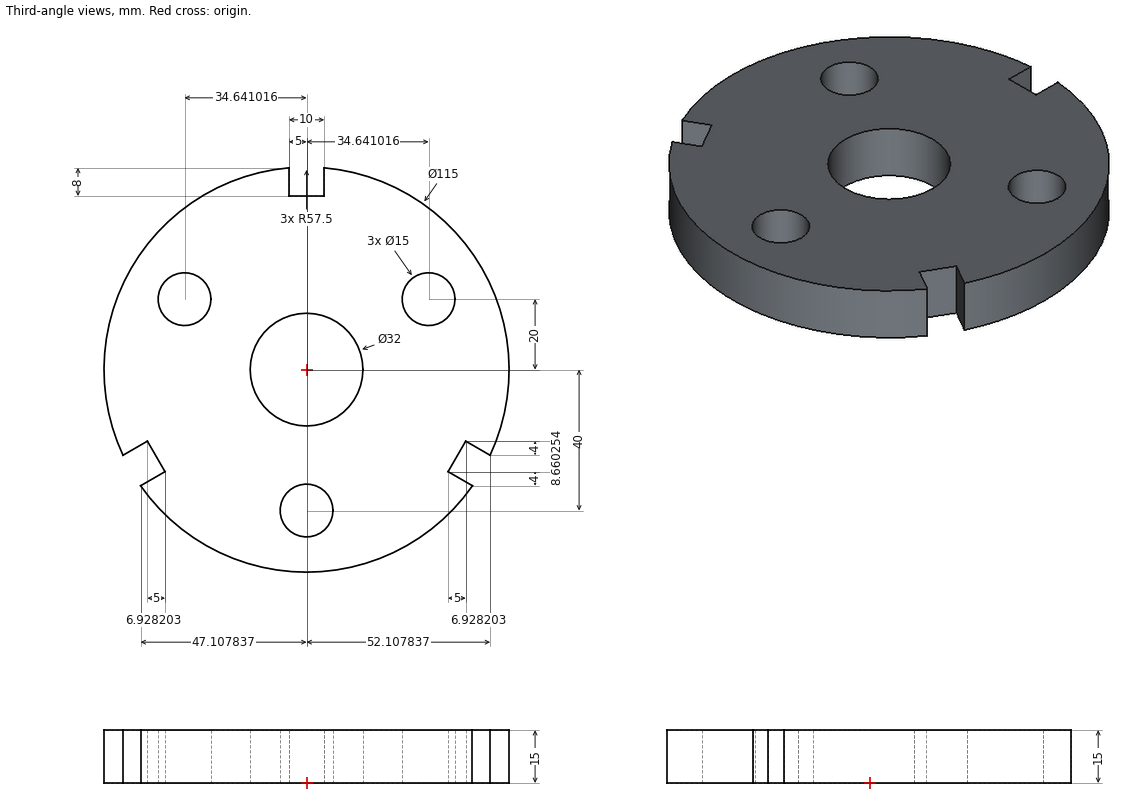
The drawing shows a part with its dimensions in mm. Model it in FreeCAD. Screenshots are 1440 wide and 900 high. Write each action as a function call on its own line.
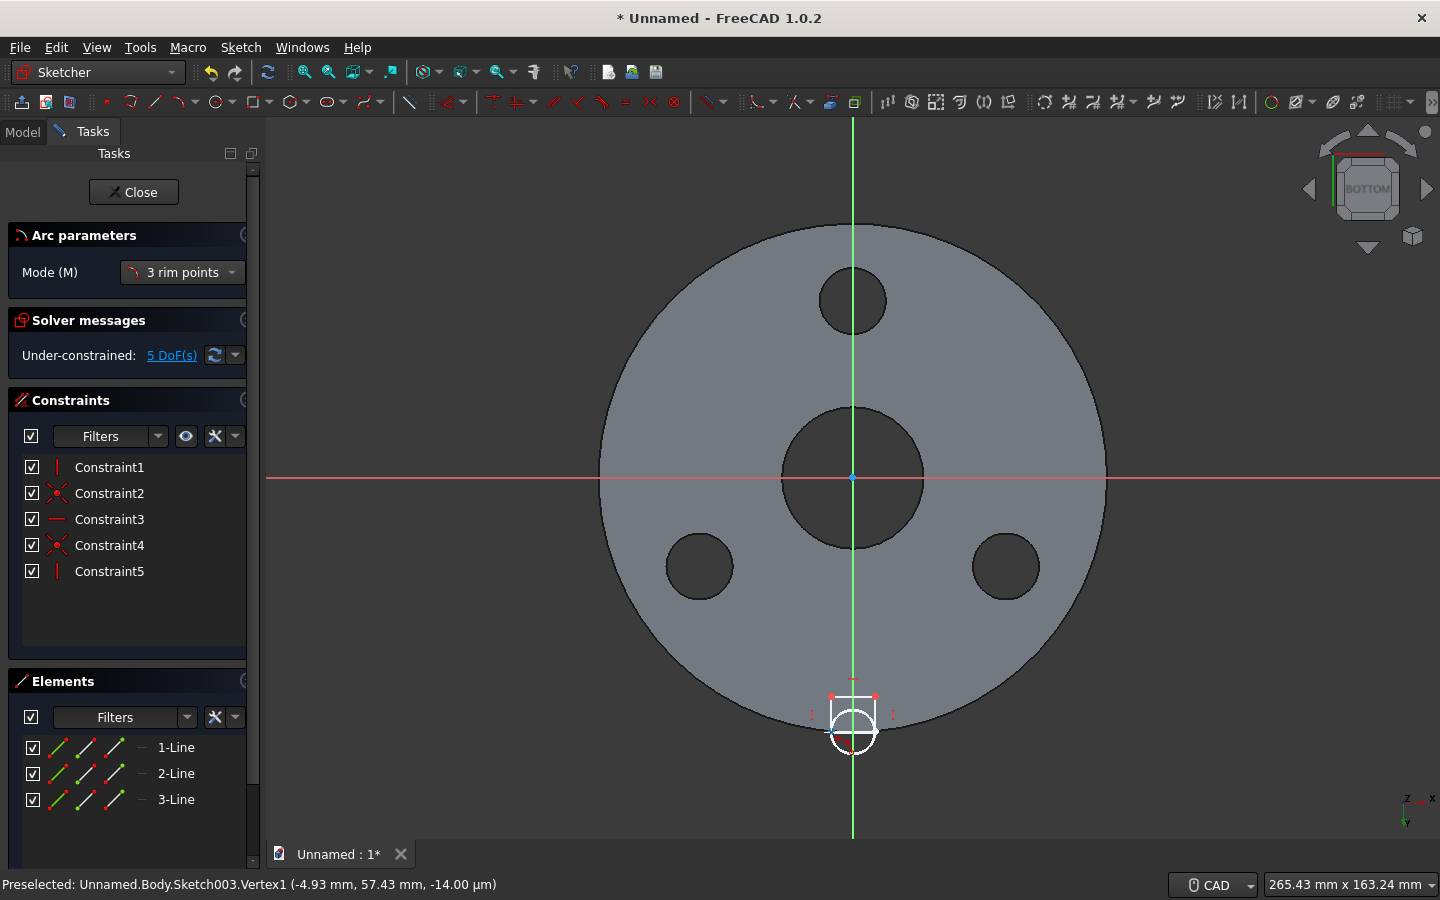
scroll(848, 732, up, 15)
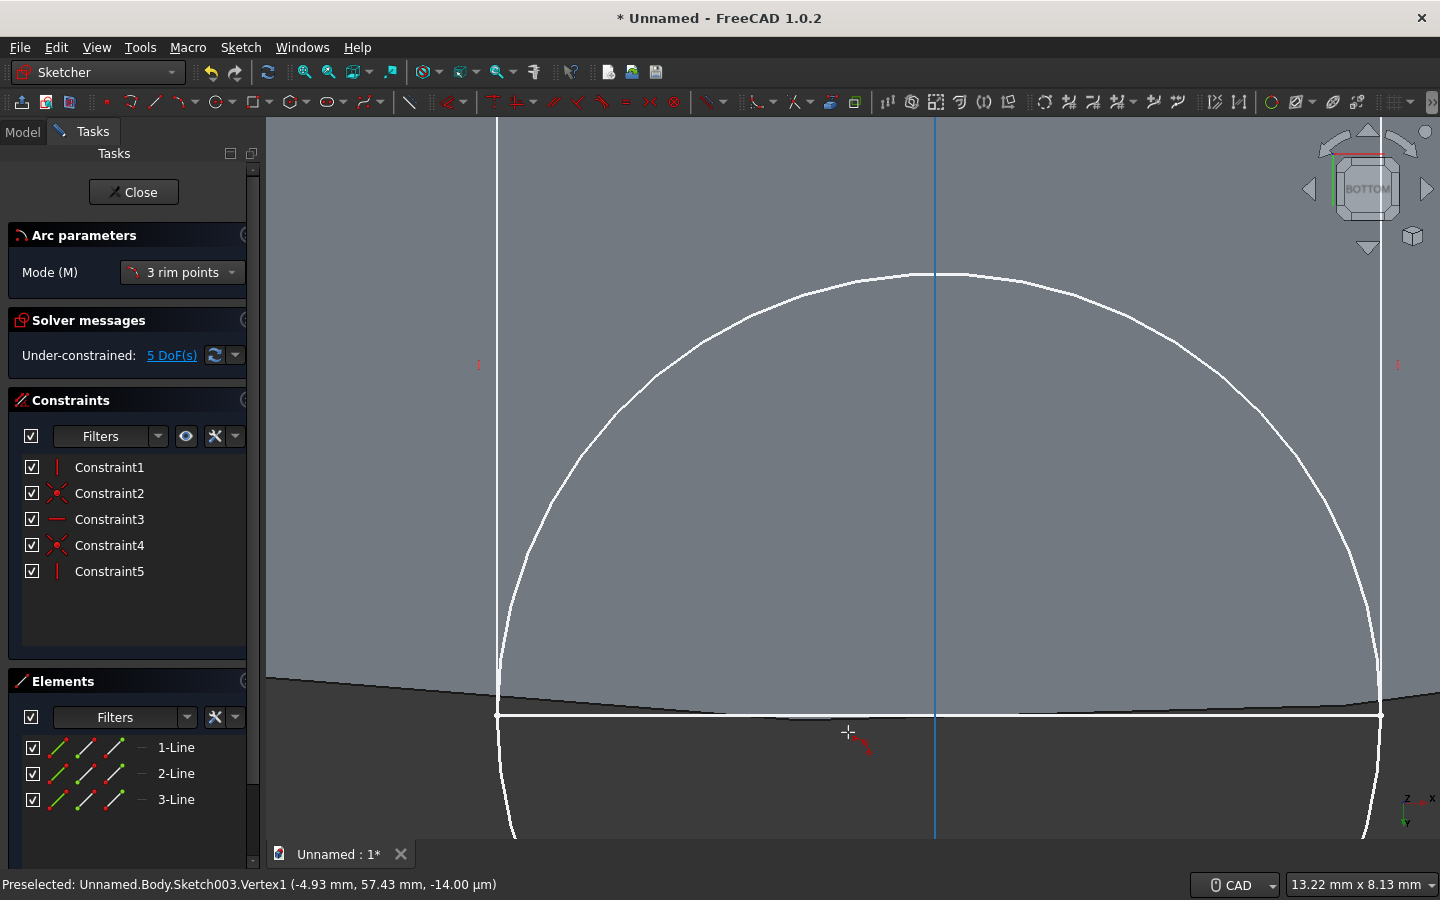
click(846, 721)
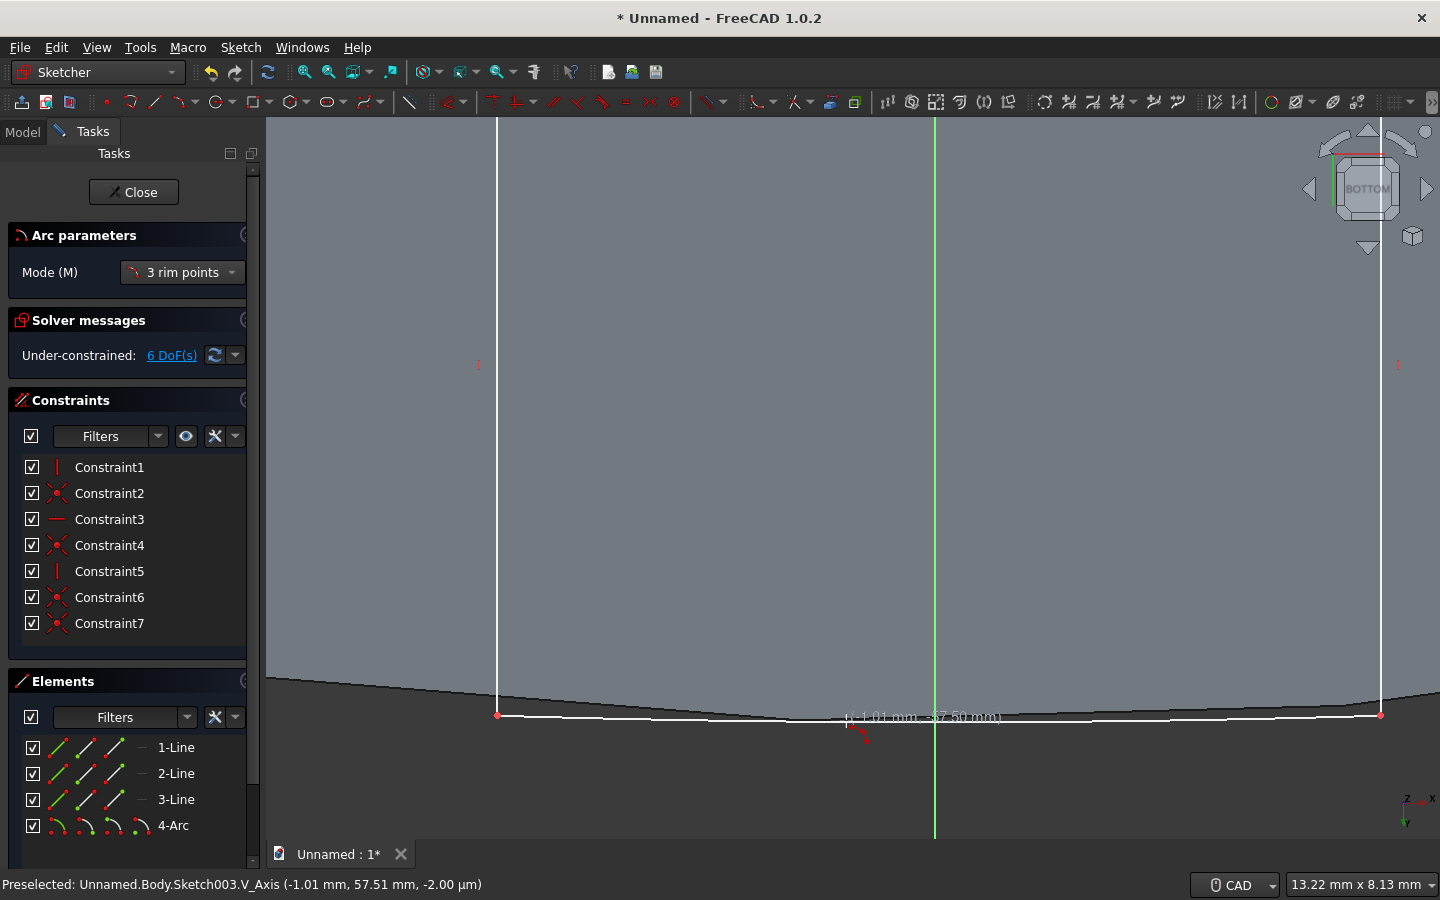
click(132, 102)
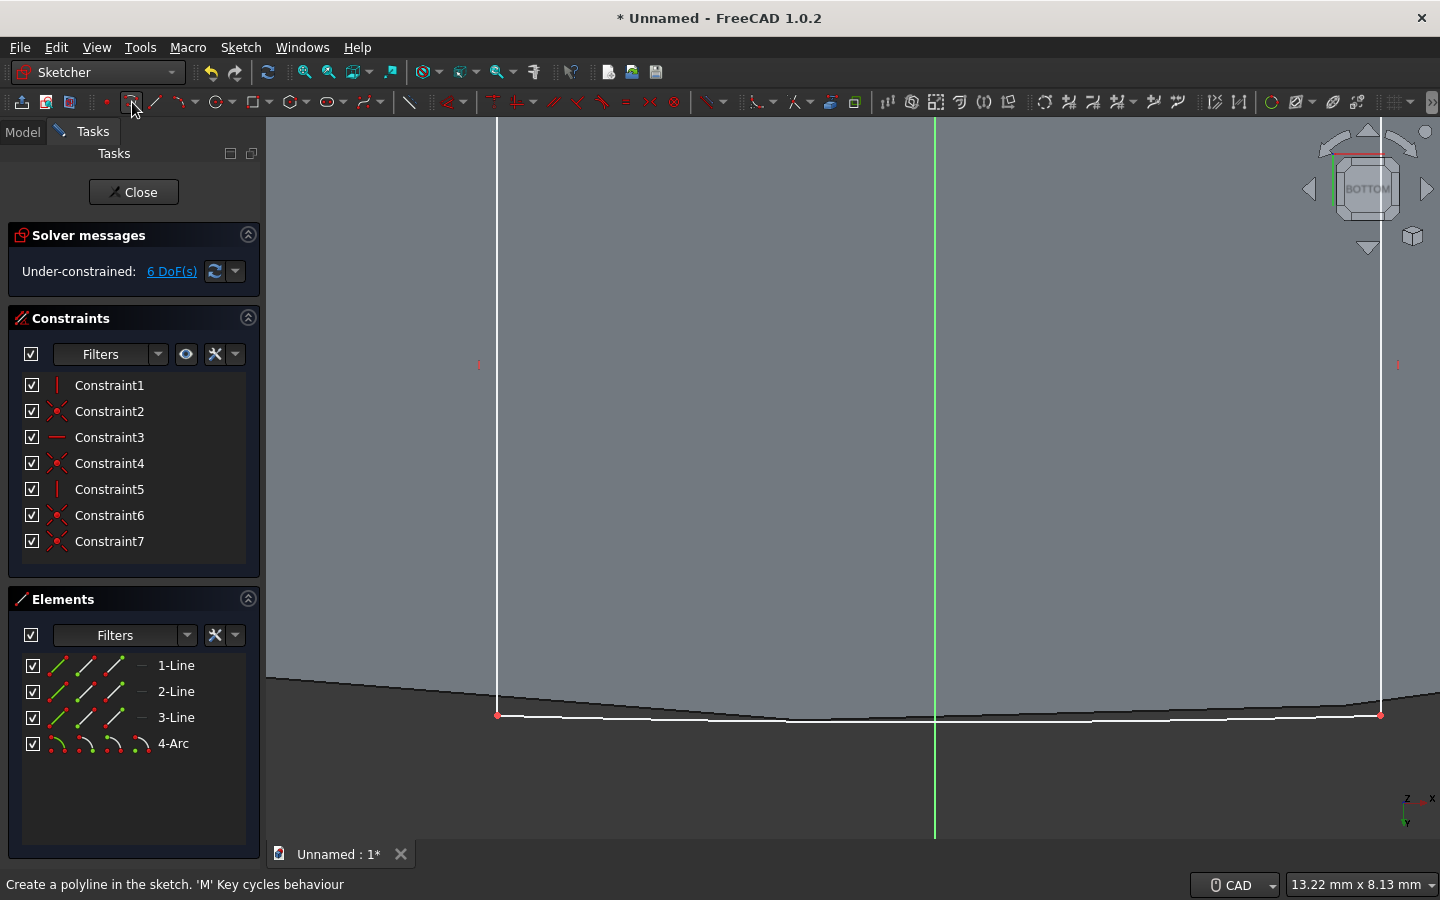
scroll(775, 722, down, 14)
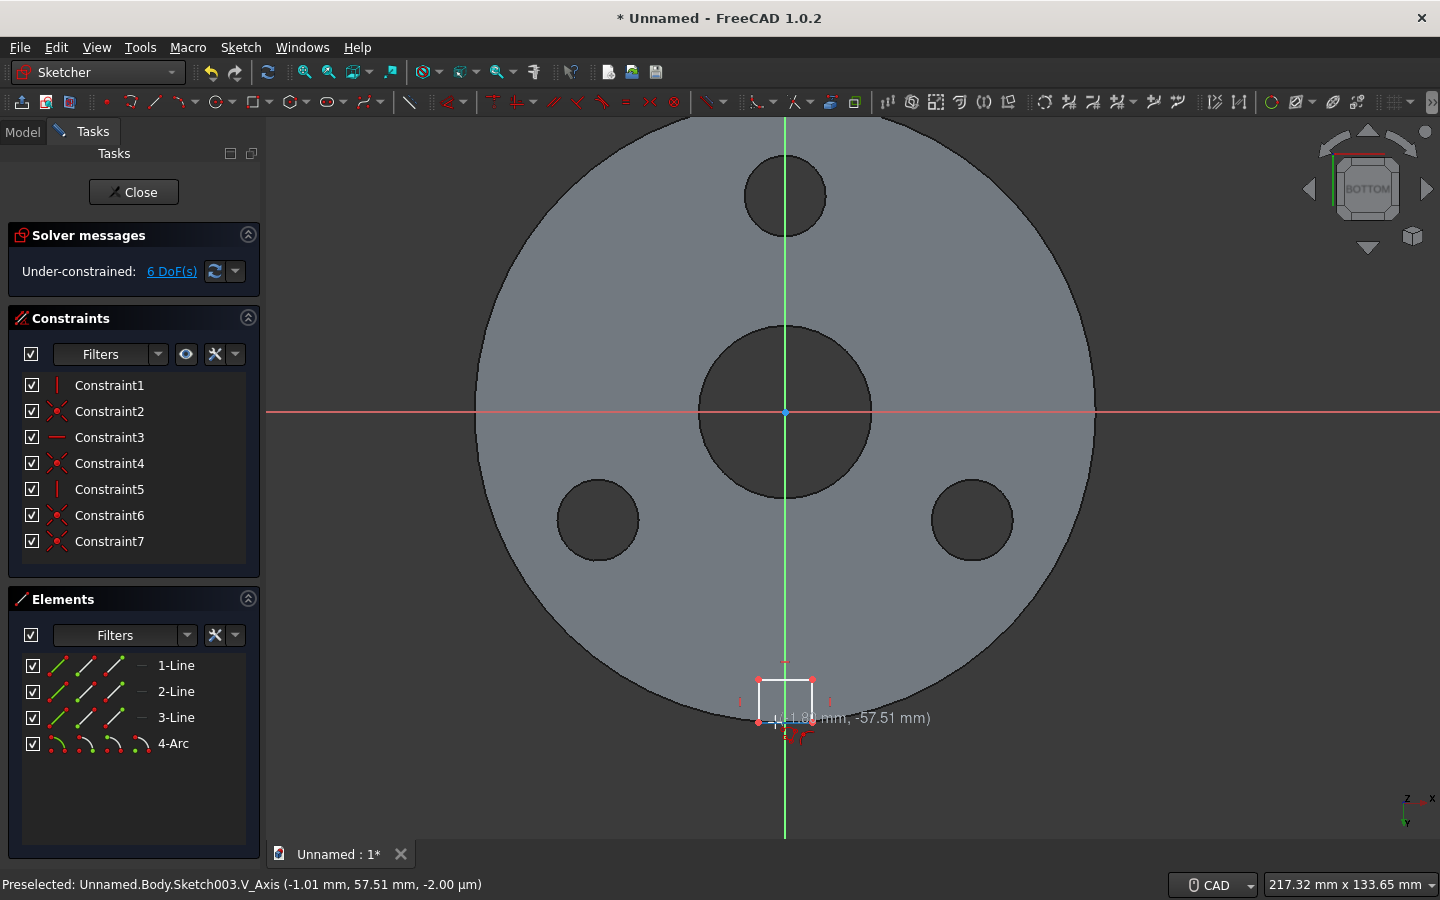
click(1067, 281)
click(1029, 302)
click(1002, 256)
click(1040, 234)
right_click(1040, 234)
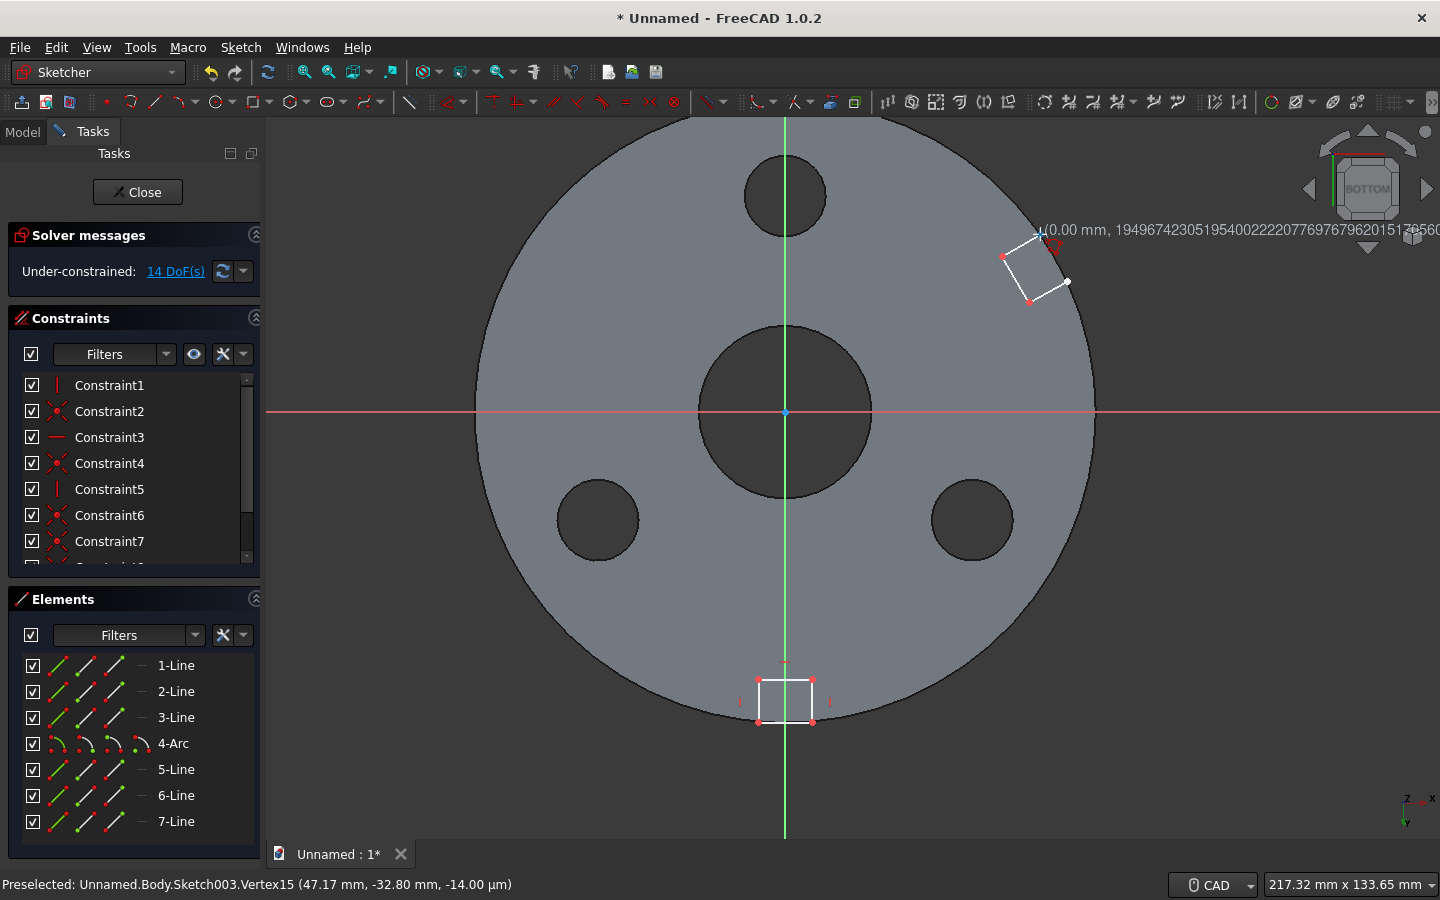
click(180, 102)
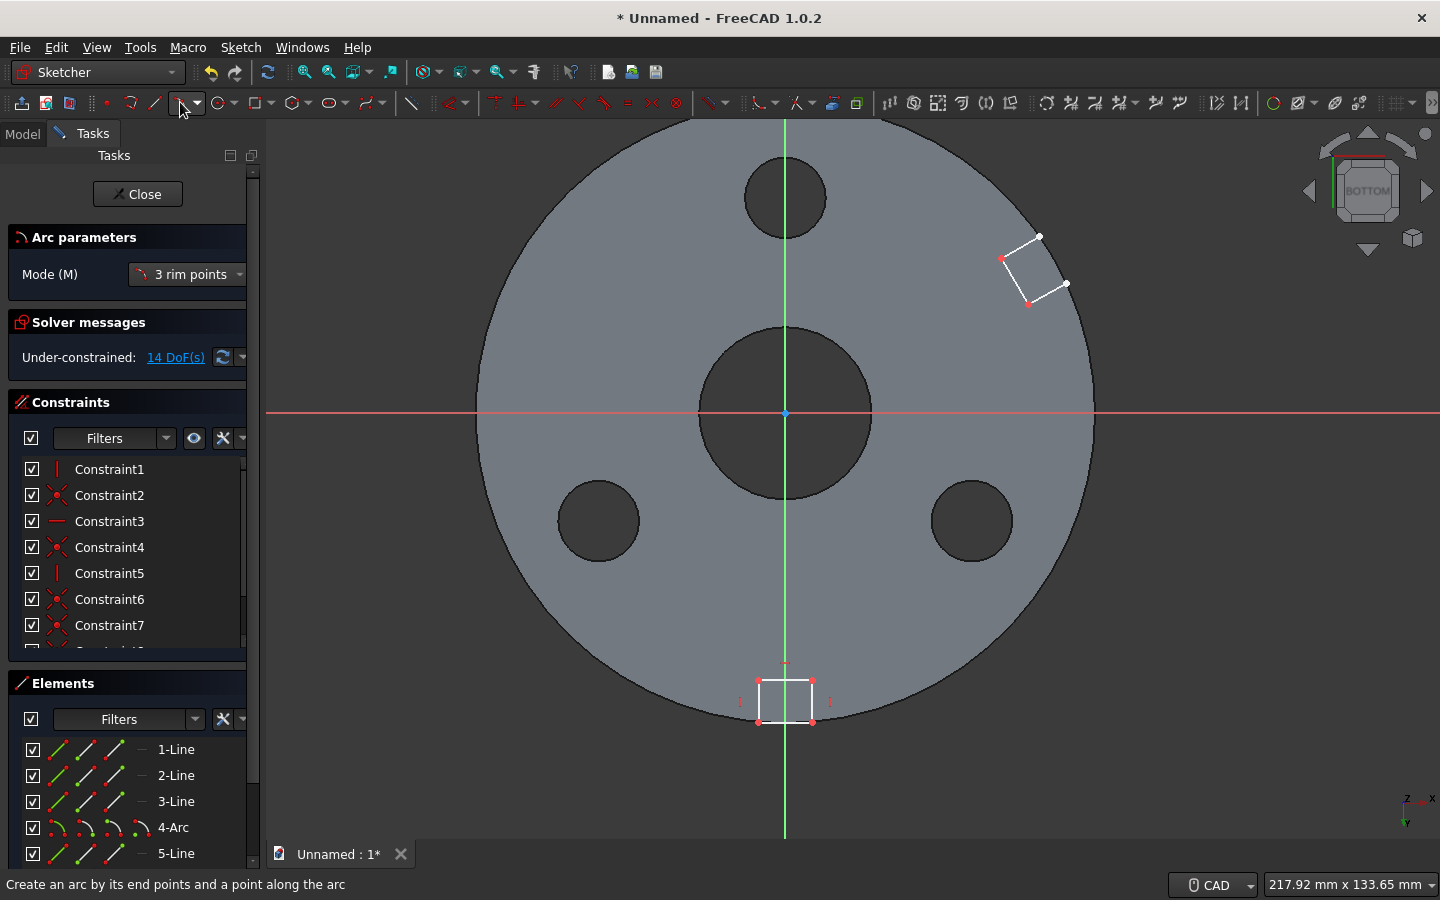
click(1039, 237)
click(1066, 284)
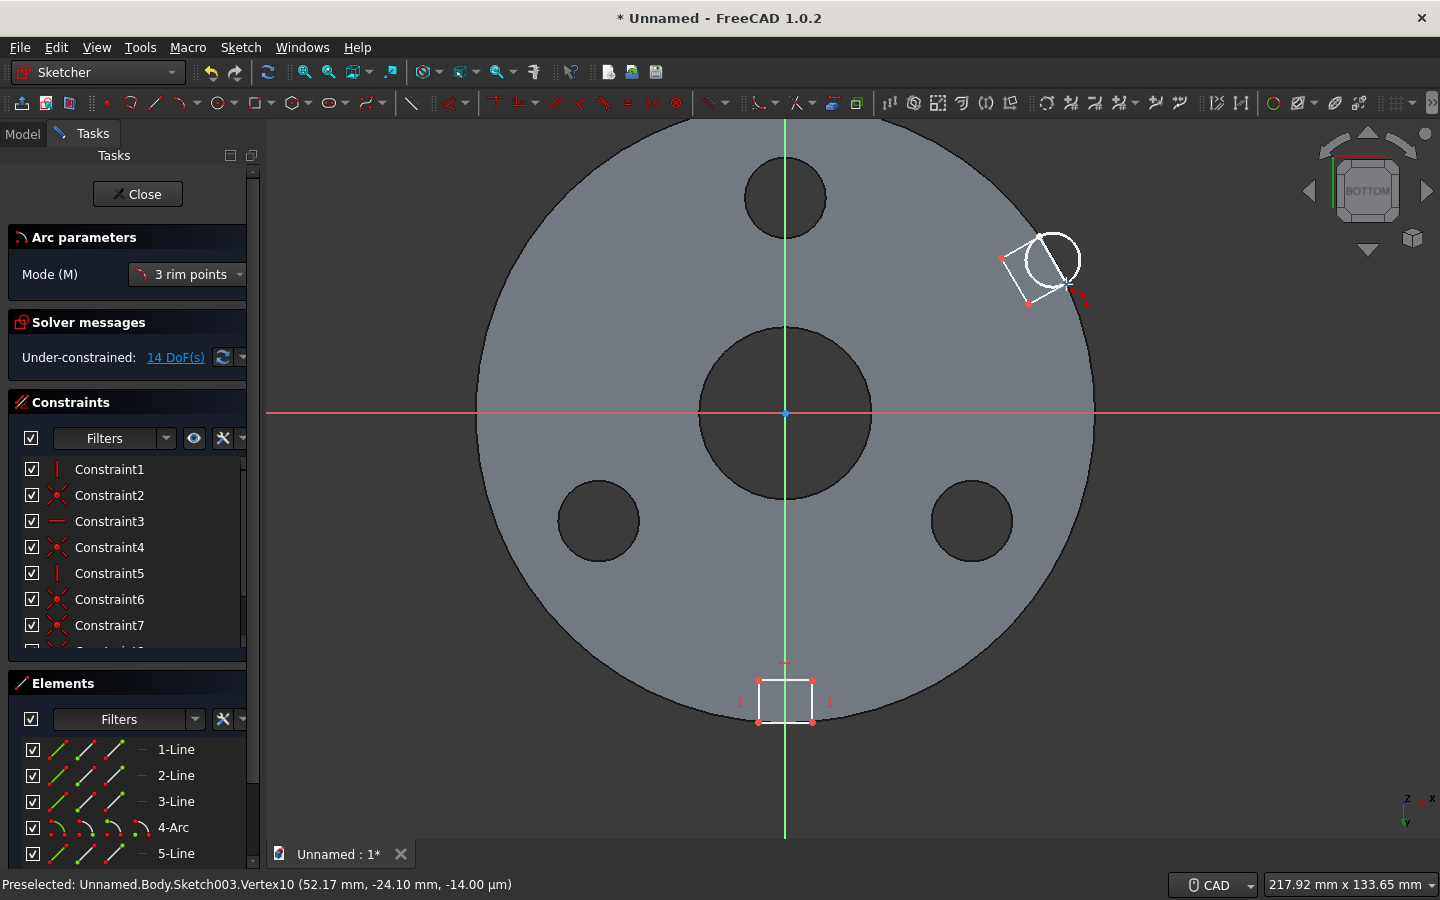
scroll(1054, 258, up, 14)